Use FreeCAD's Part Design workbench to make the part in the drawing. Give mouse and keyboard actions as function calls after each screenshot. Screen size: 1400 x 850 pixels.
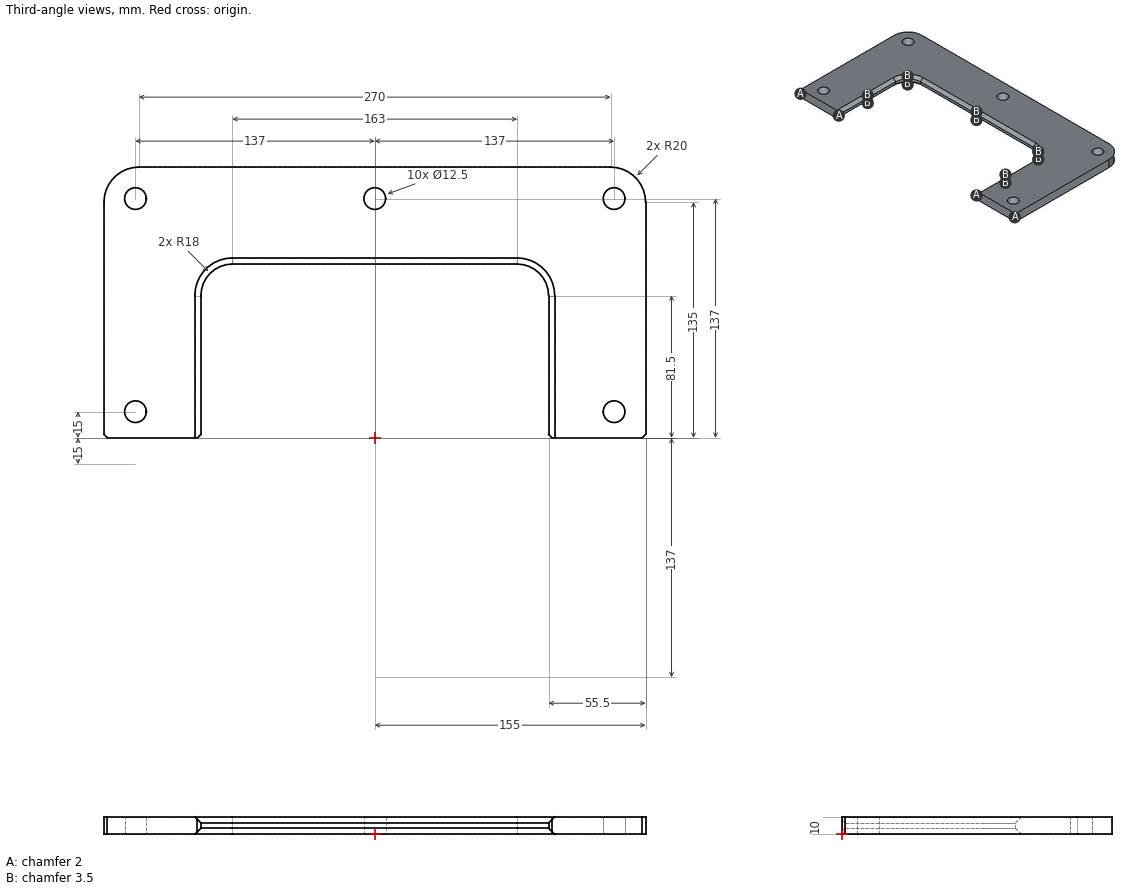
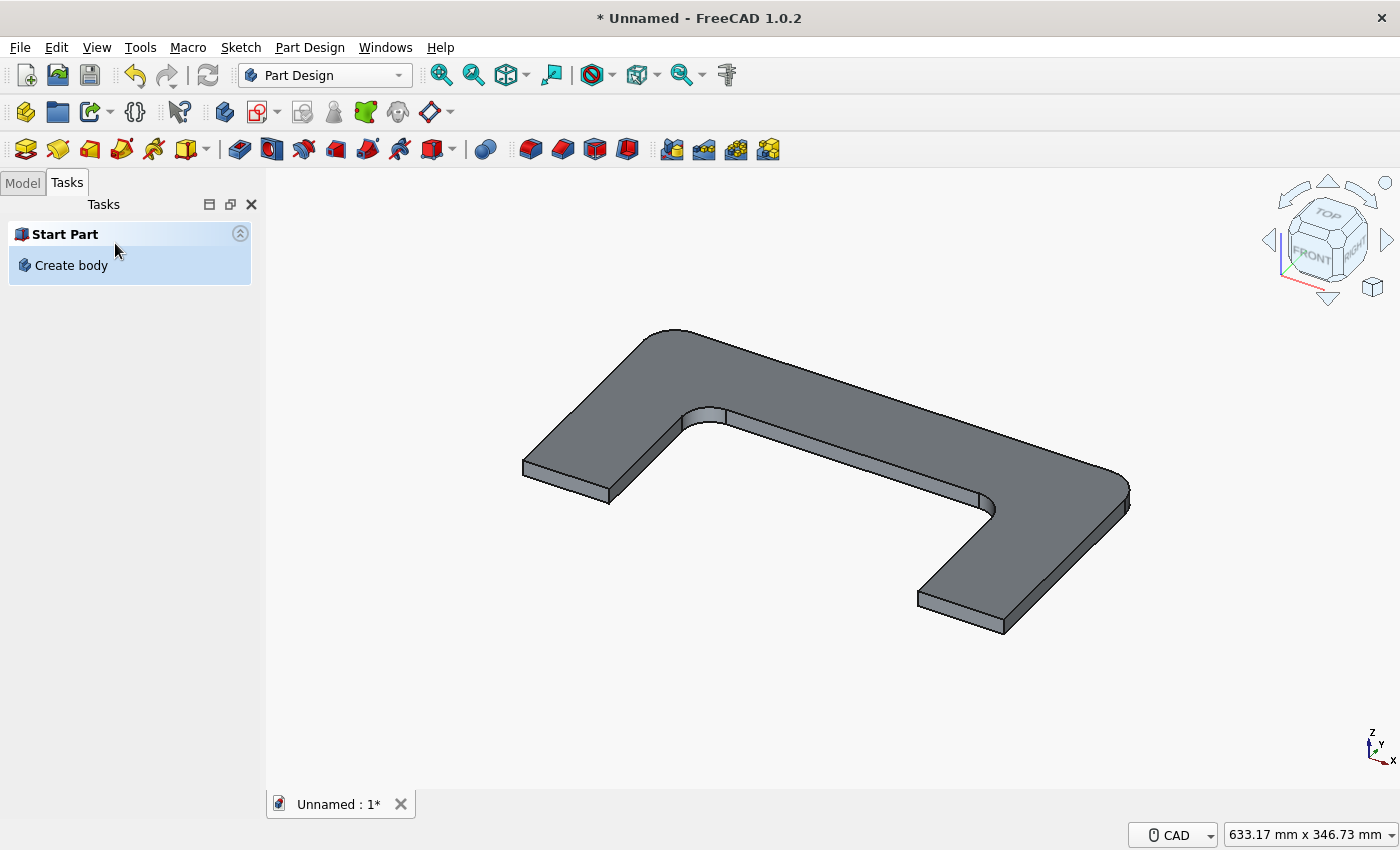
click(1010, 476)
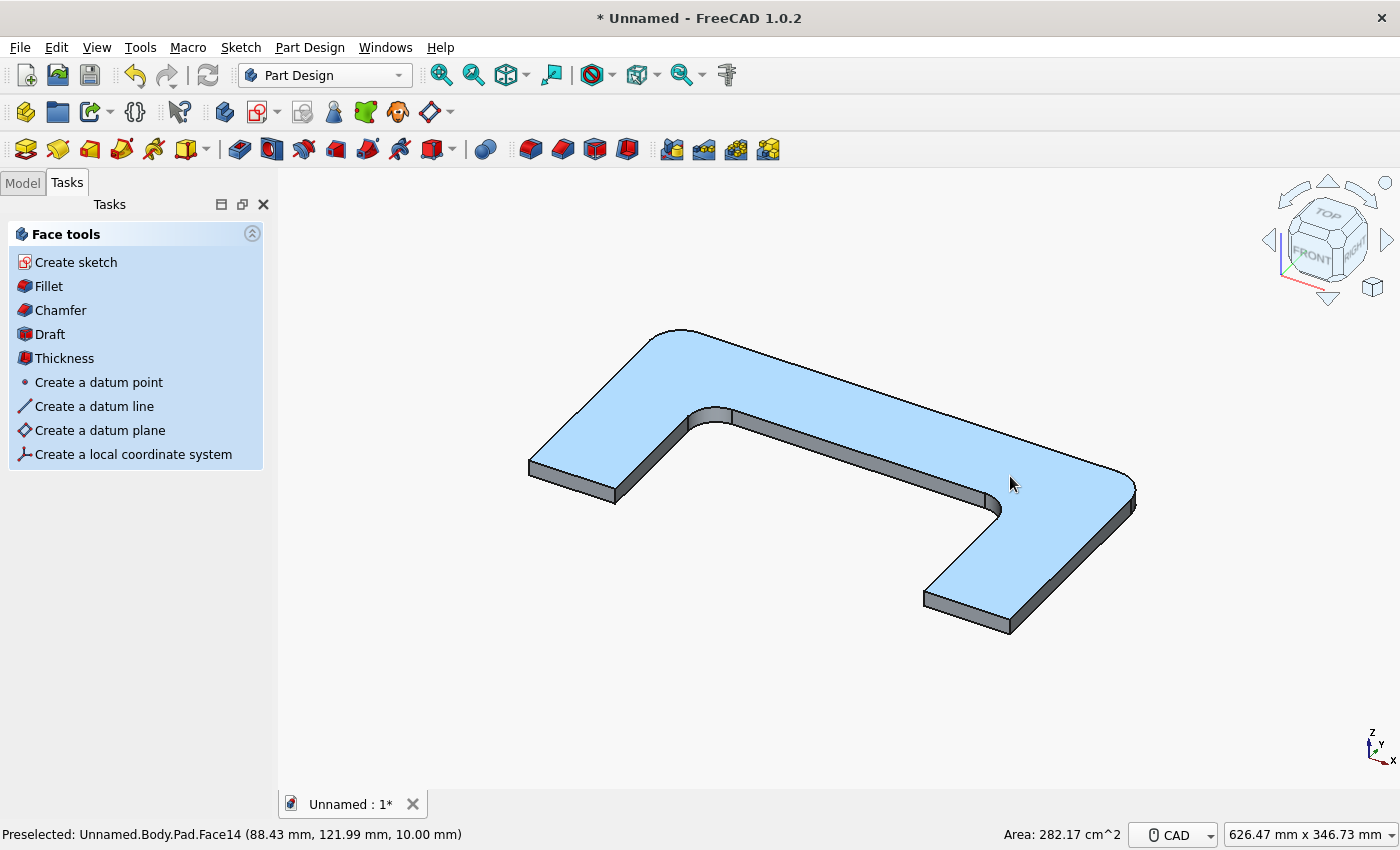
click(258, 112)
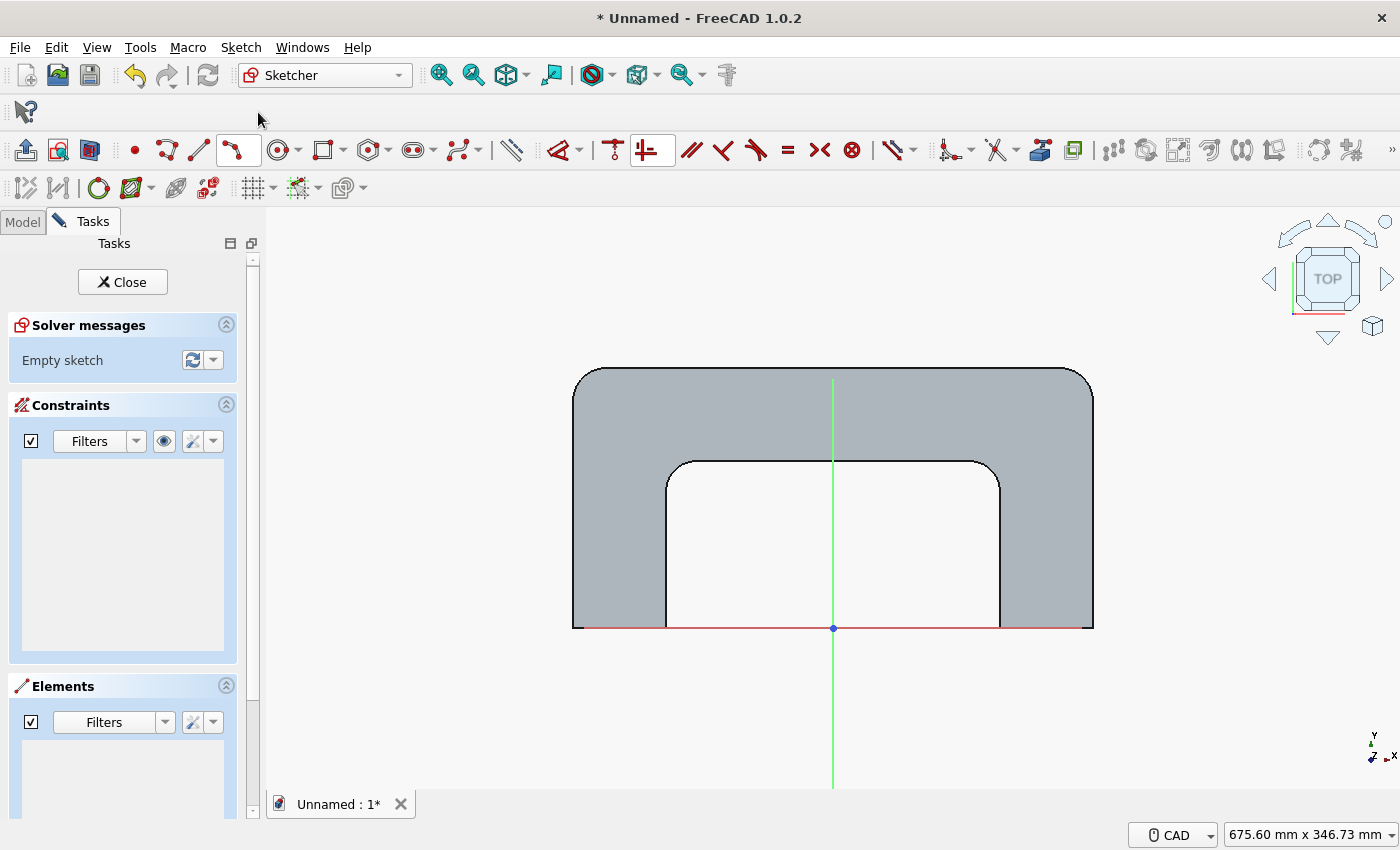
scroll(625, 235, down, 2)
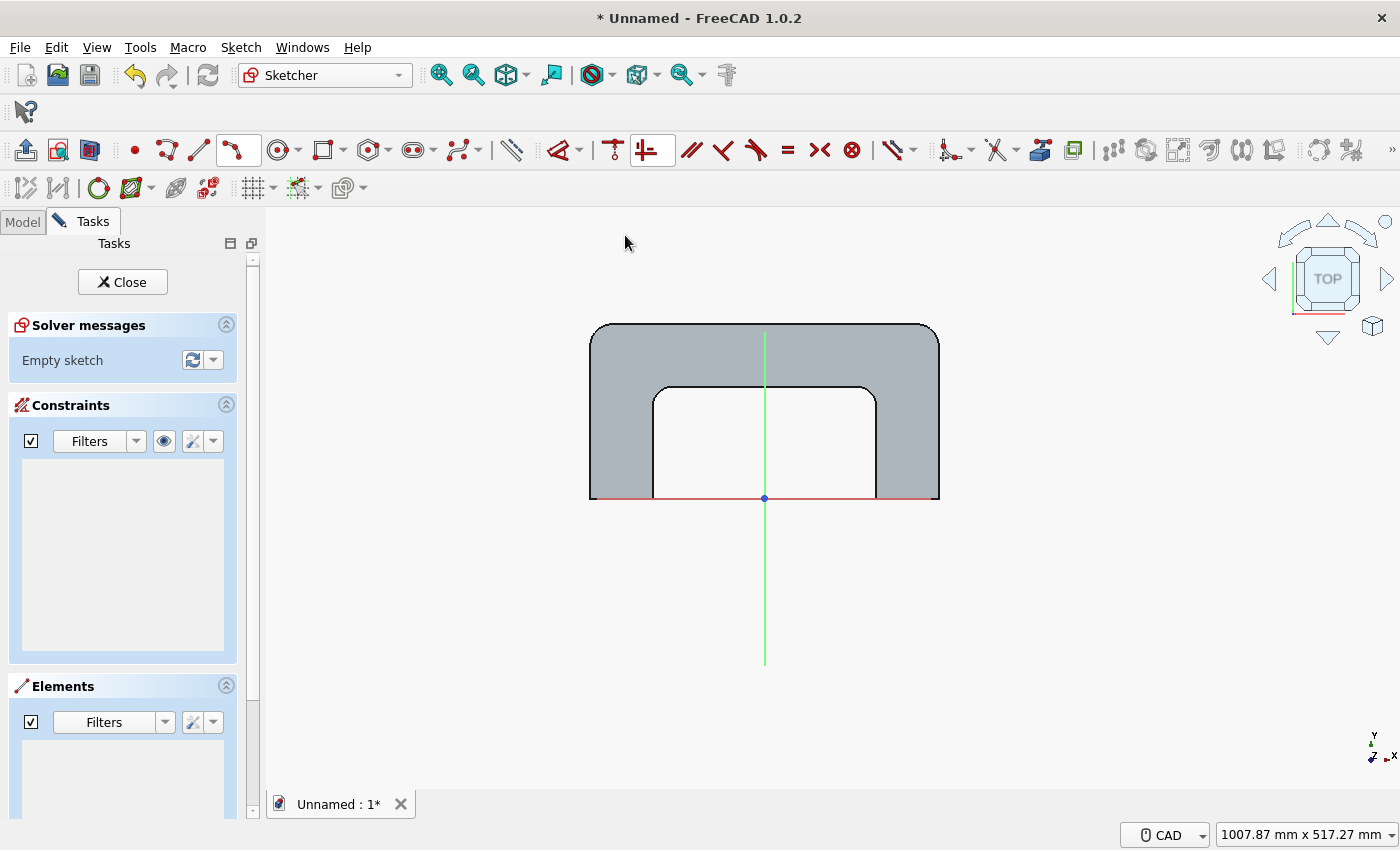
click(278, 150)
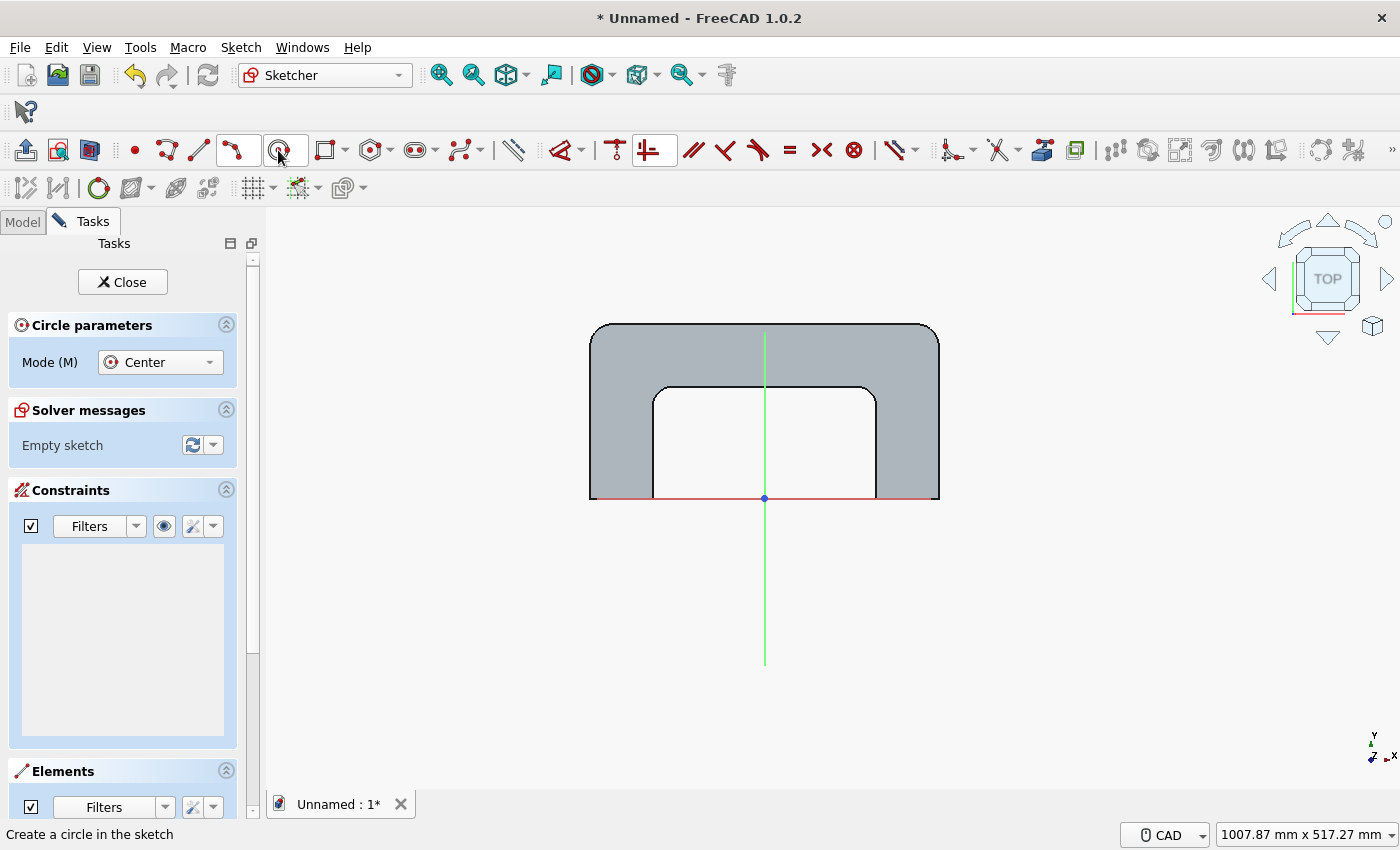
scroll(765, 344, up, 6)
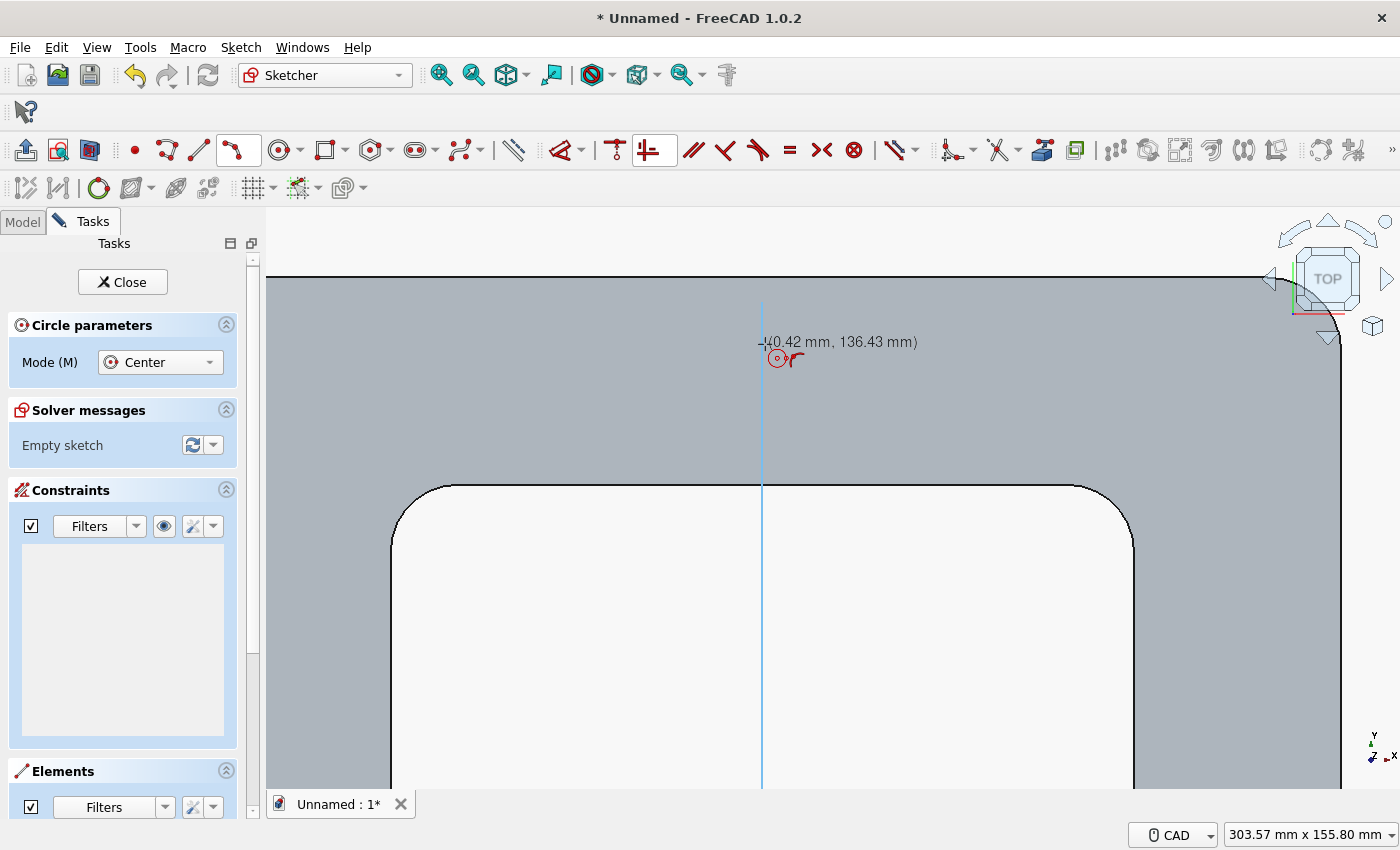
click(762, 345)
move(779, 328)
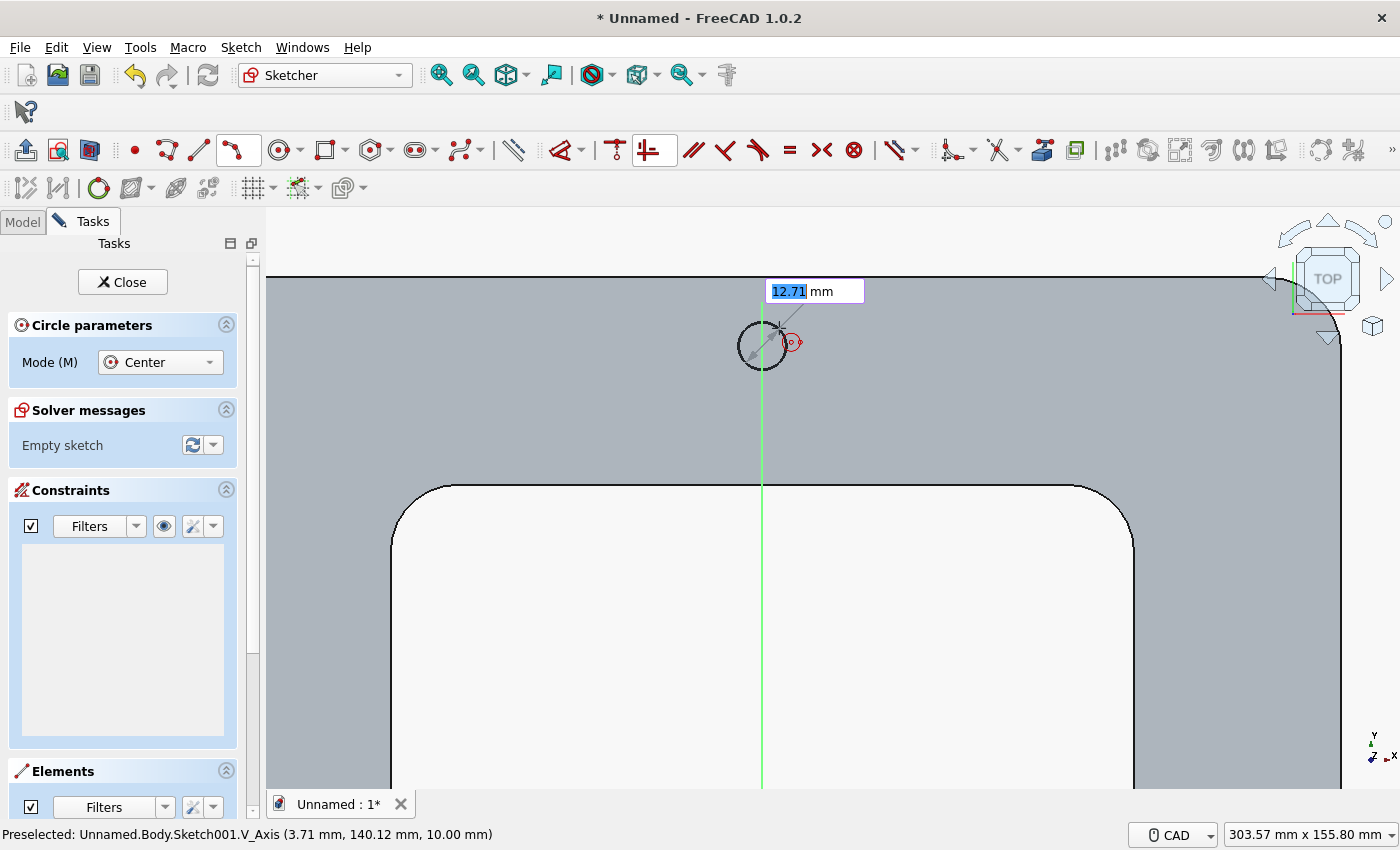
text(12.5)
key(Return)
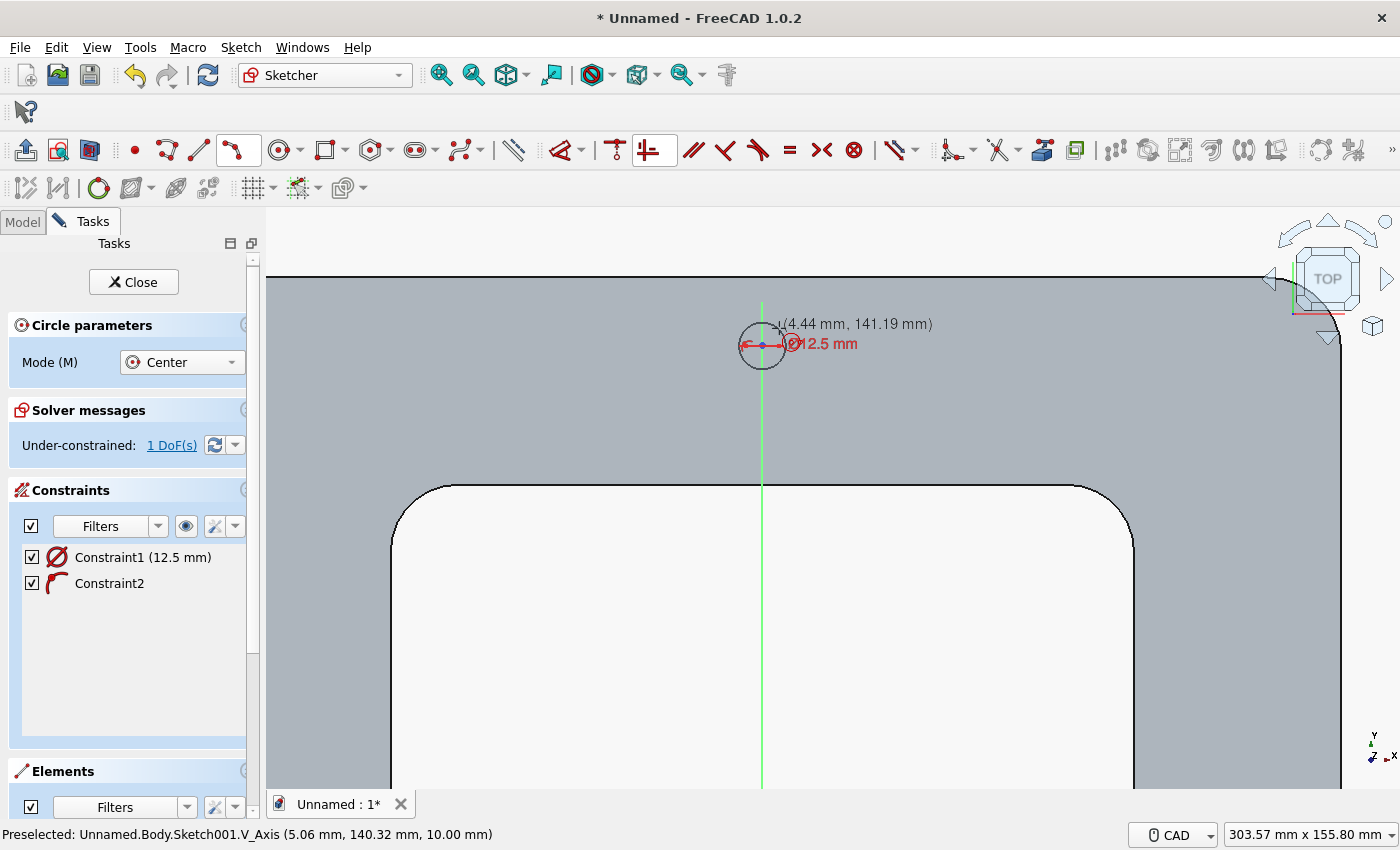
scroll(766, 289, down, 5)